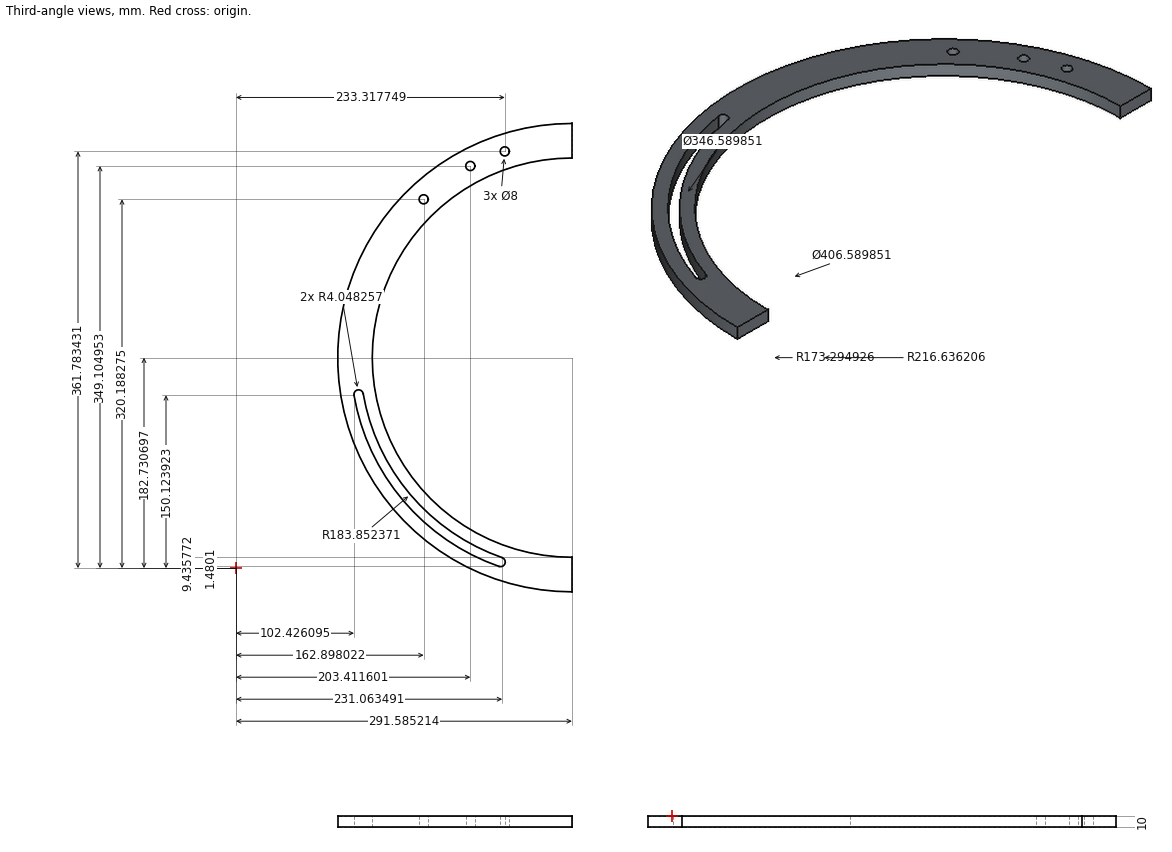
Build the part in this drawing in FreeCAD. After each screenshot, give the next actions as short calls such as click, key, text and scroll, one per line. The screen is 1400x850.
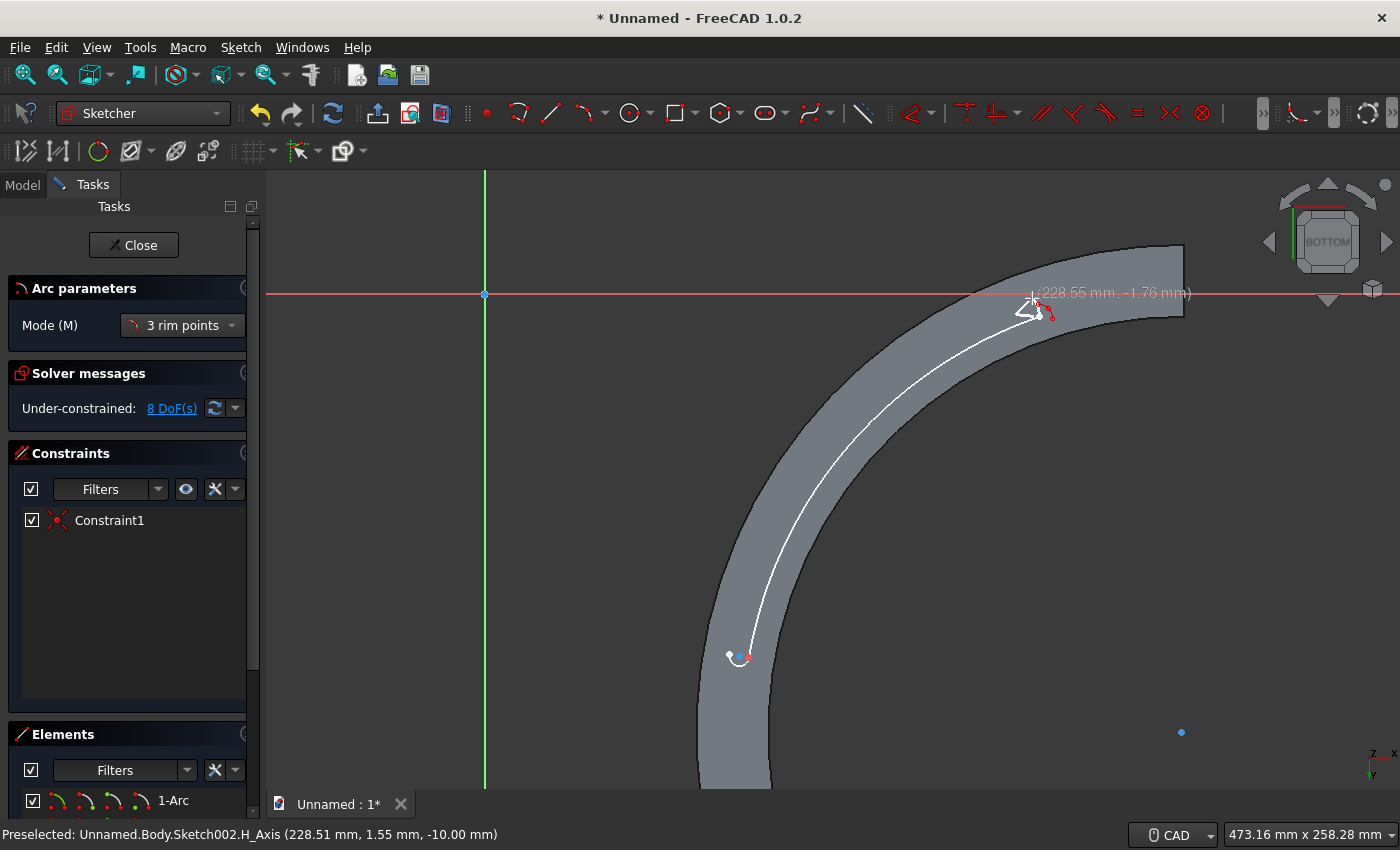
scroll(1045, 304, up, 3)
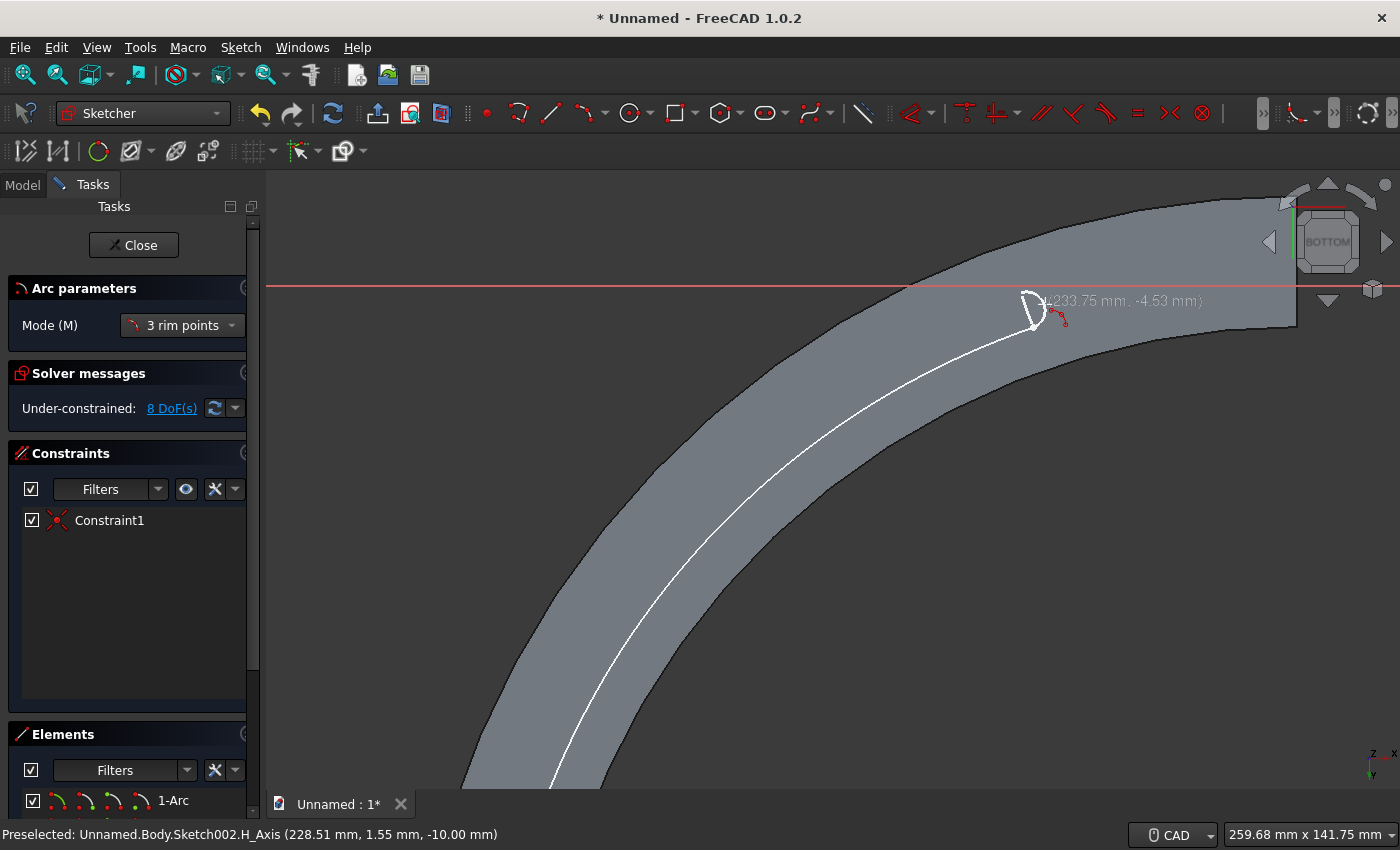
click(1044, 303)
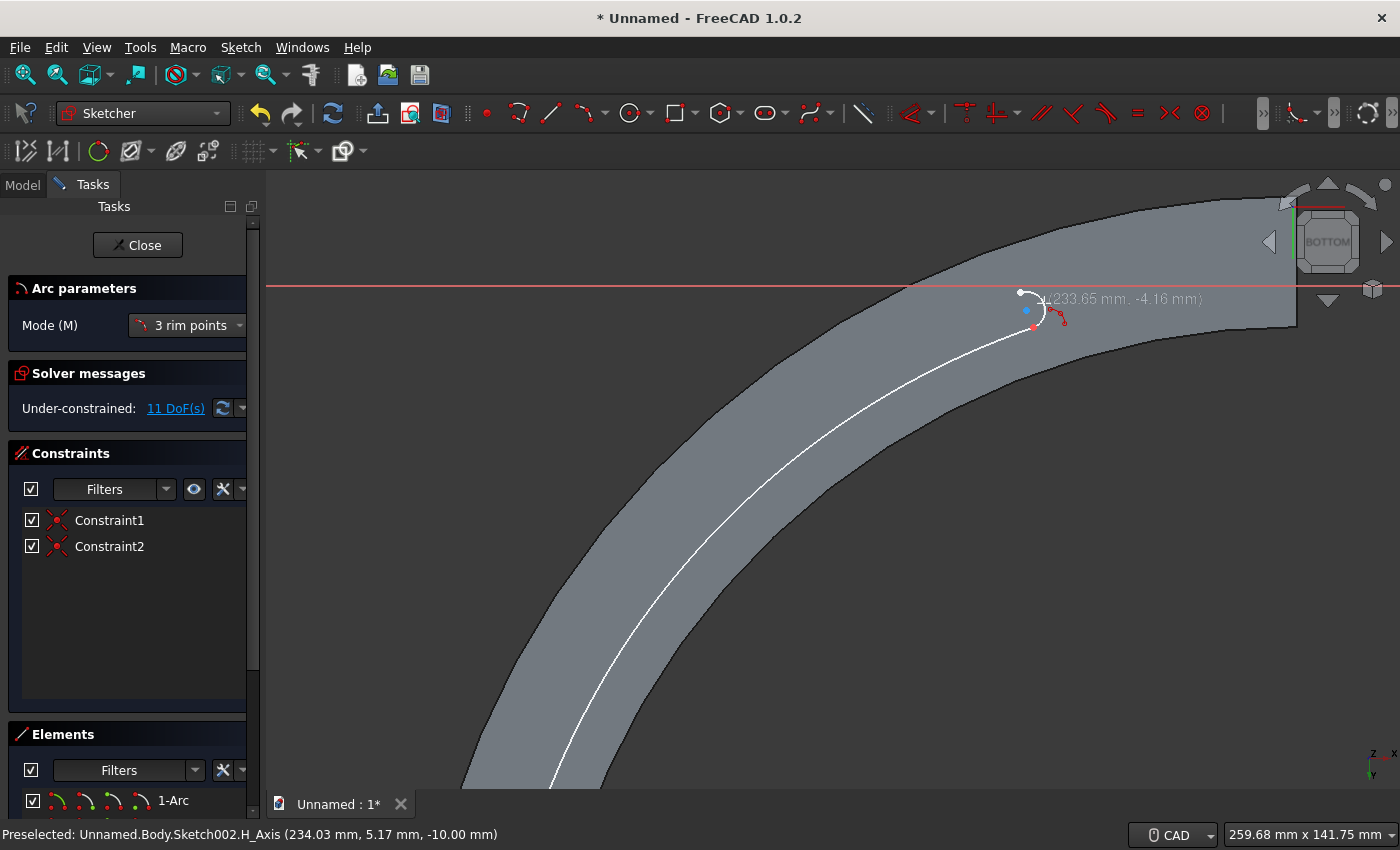
scroll(1021, 292, up, 5)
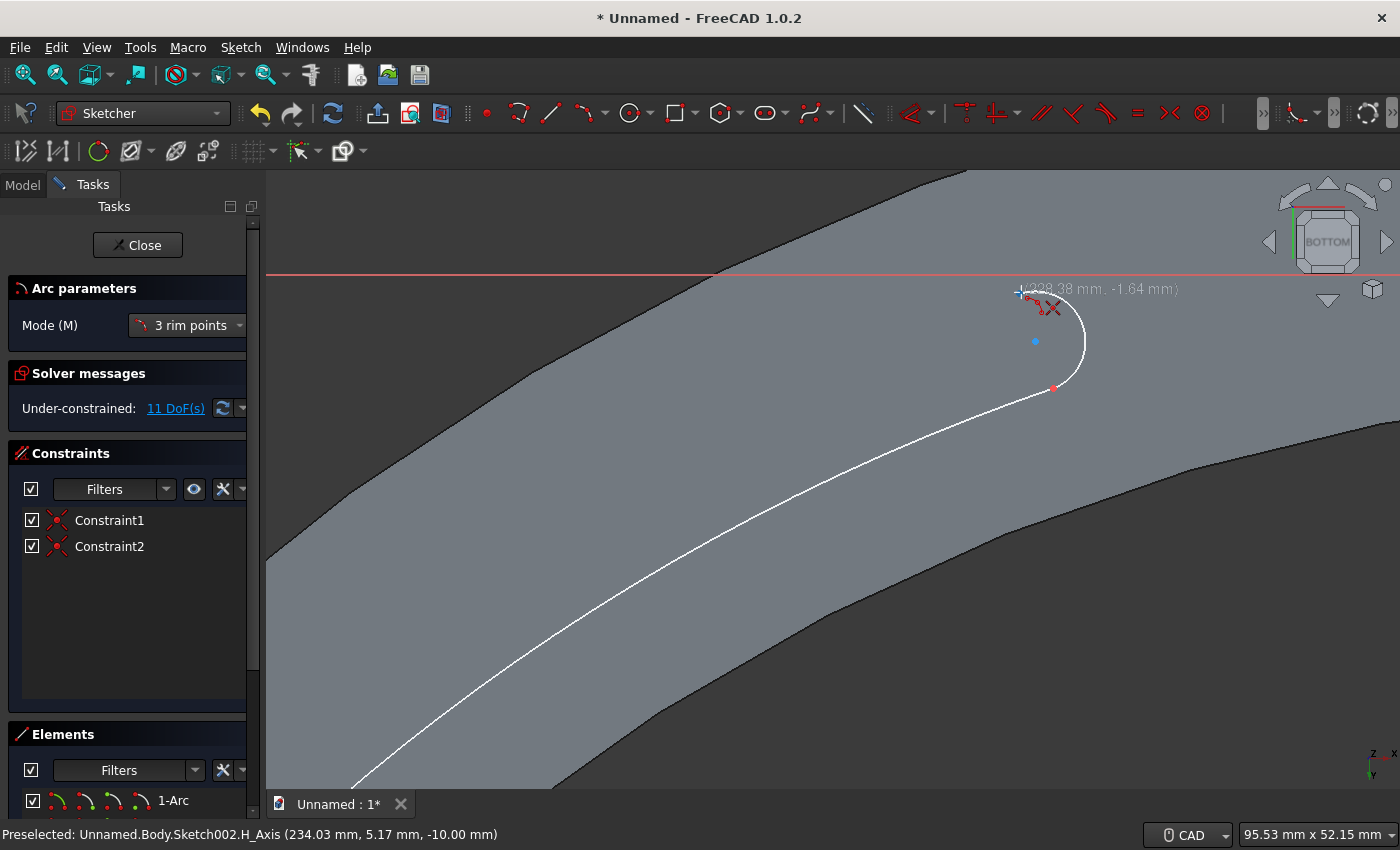
click(1020, 294)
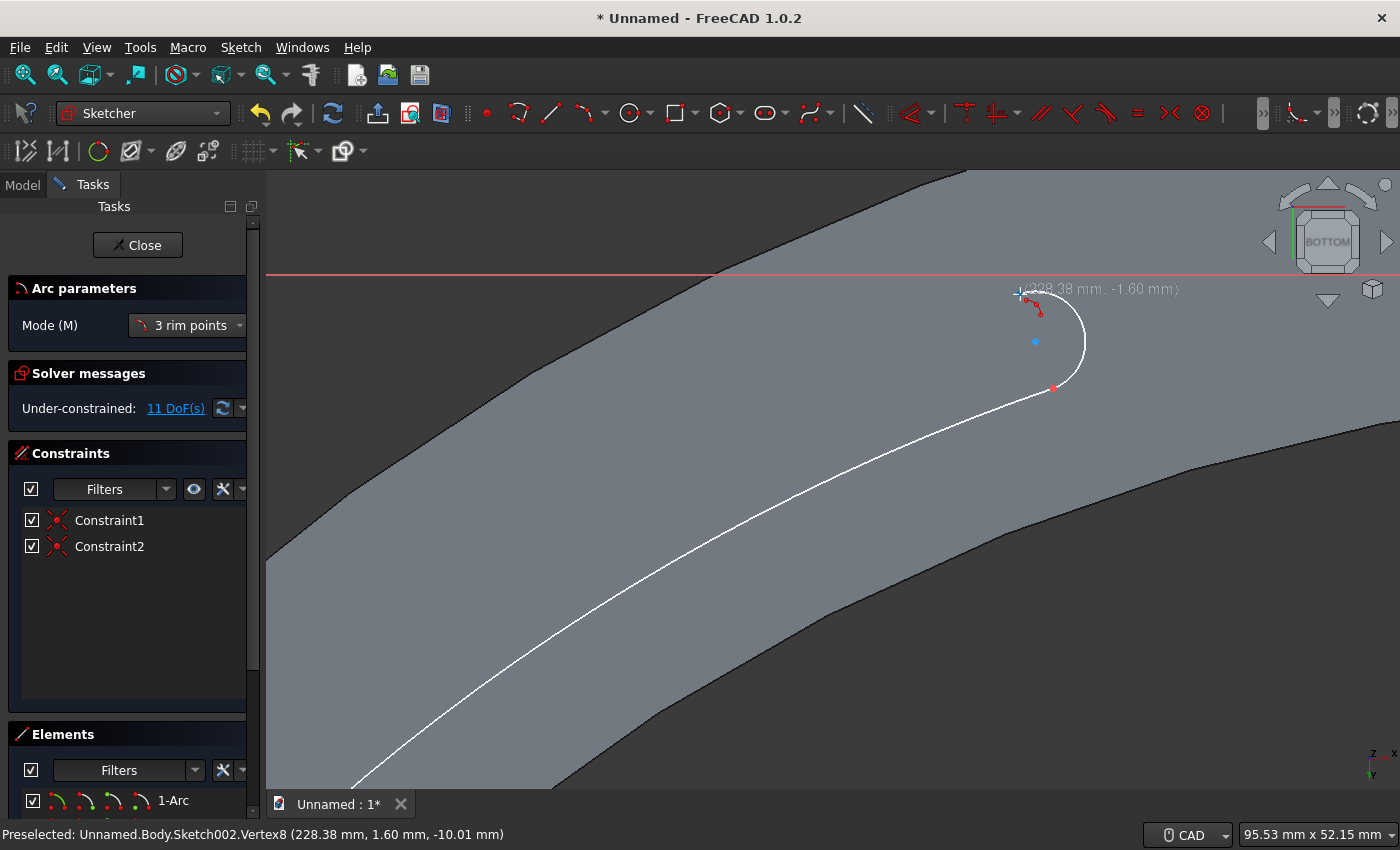
scroll(1035, 299, down, 8)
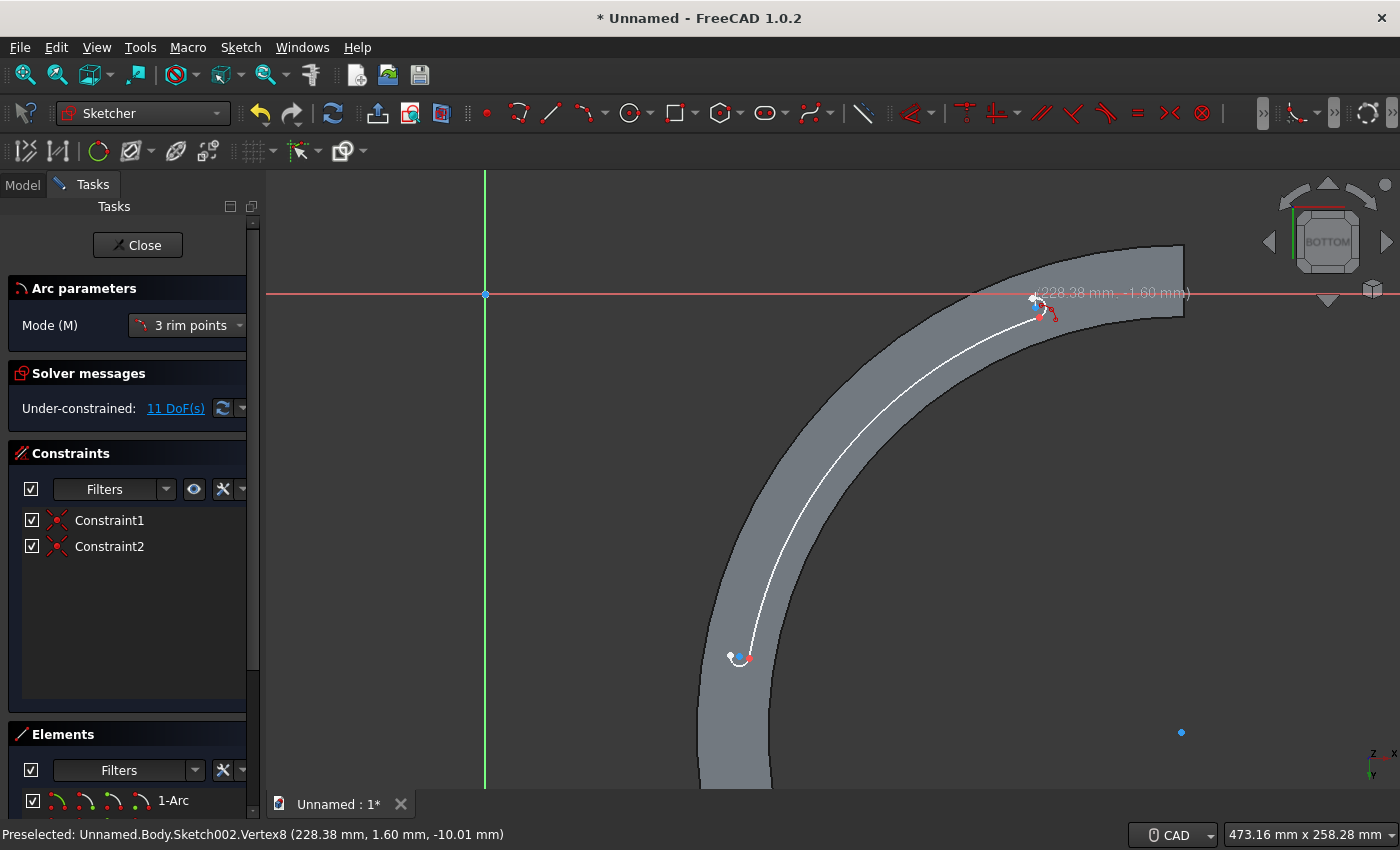
scroll(731, 654, up, 3)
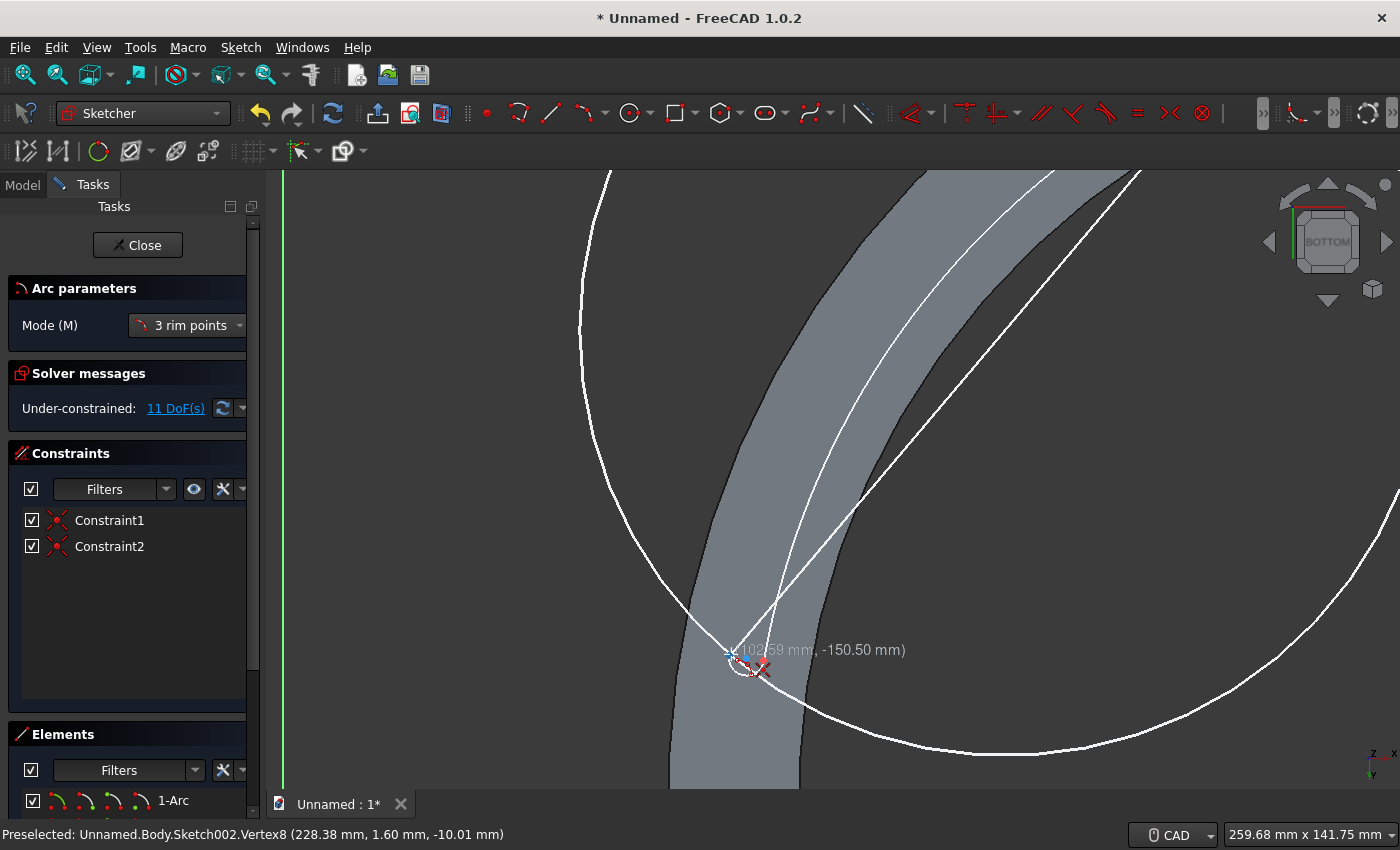
click(729, 655)
click(917, 254)
key(Escape)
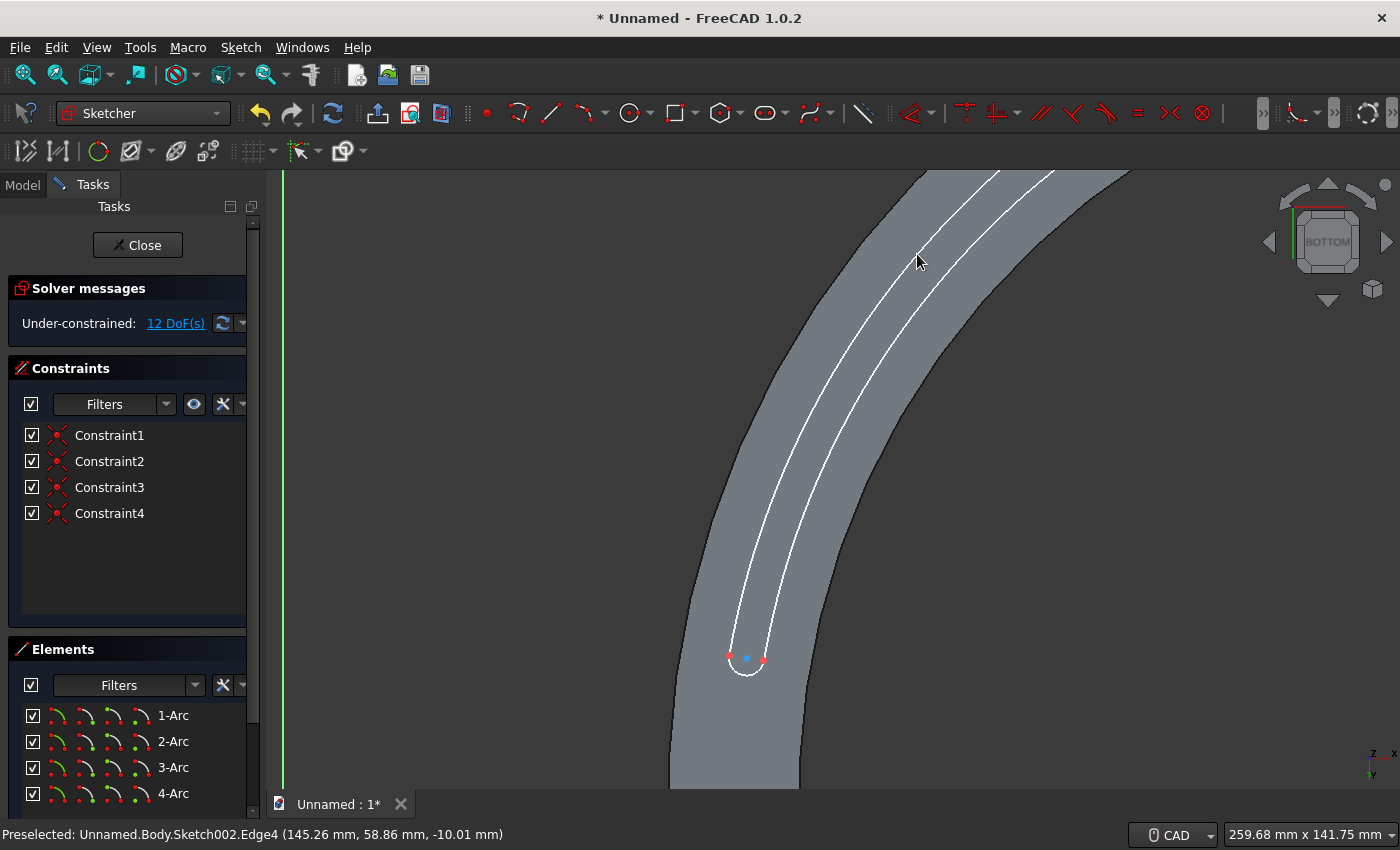
click(734, 670)